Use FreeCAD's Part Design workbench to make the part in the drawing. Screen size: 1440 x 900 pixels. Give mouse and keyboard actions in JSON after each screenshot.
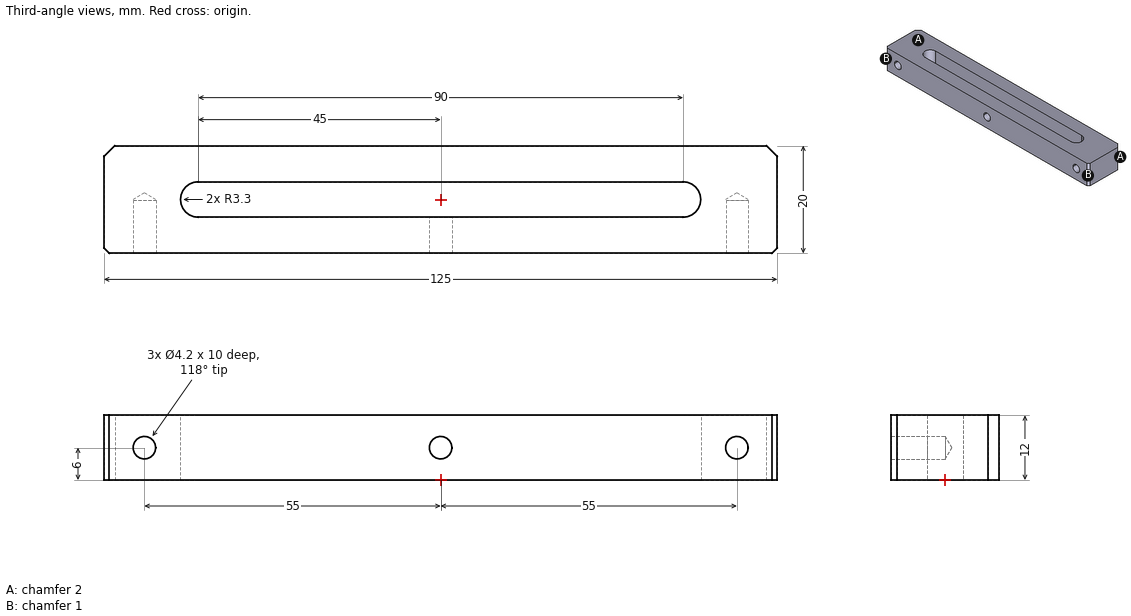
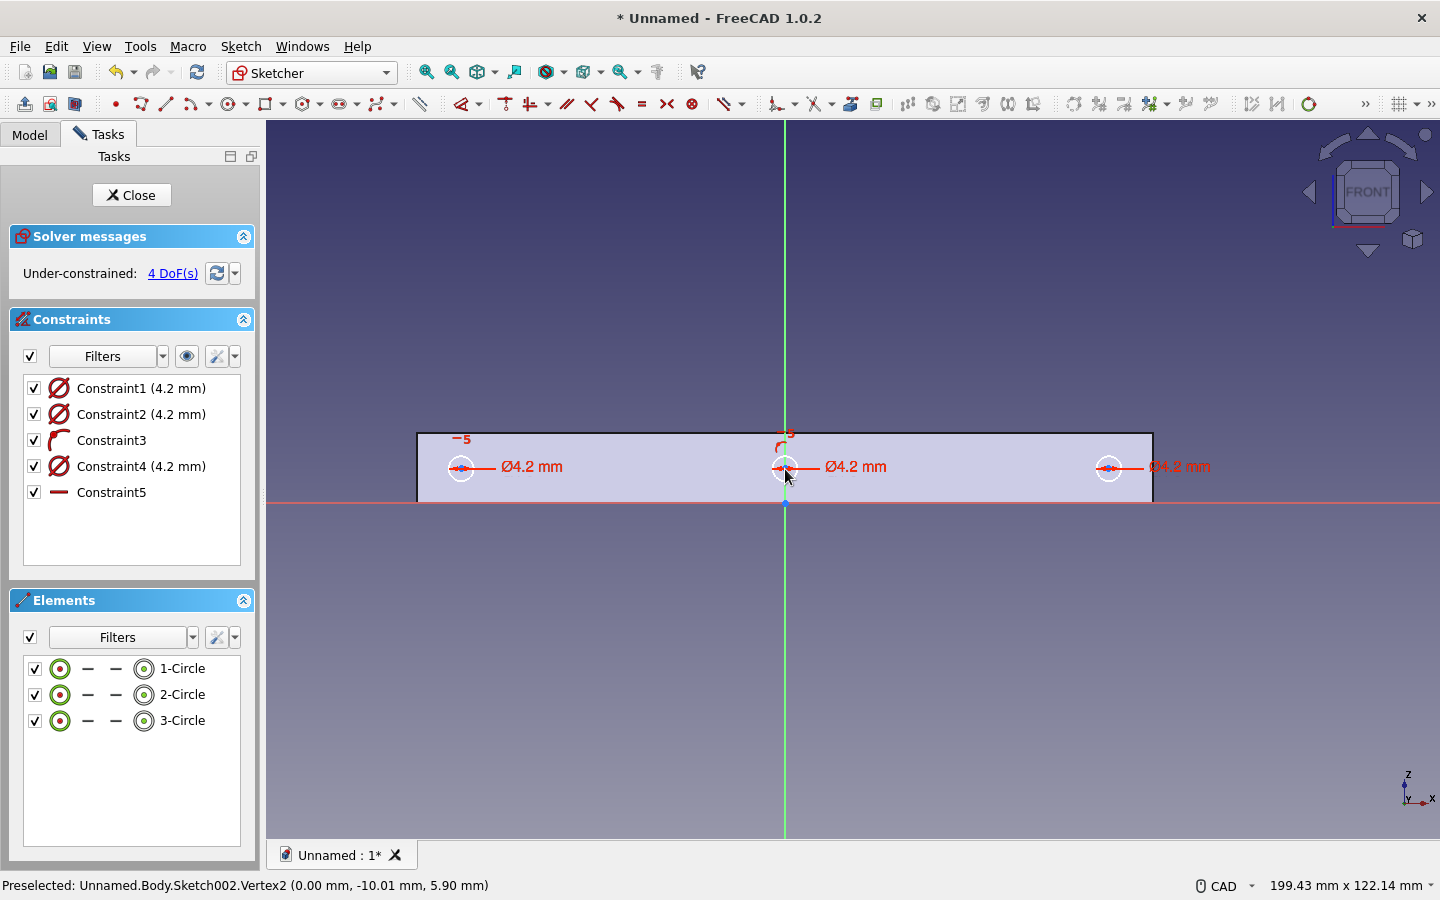
{"action": "left_click", "coordinate": [785, 469]}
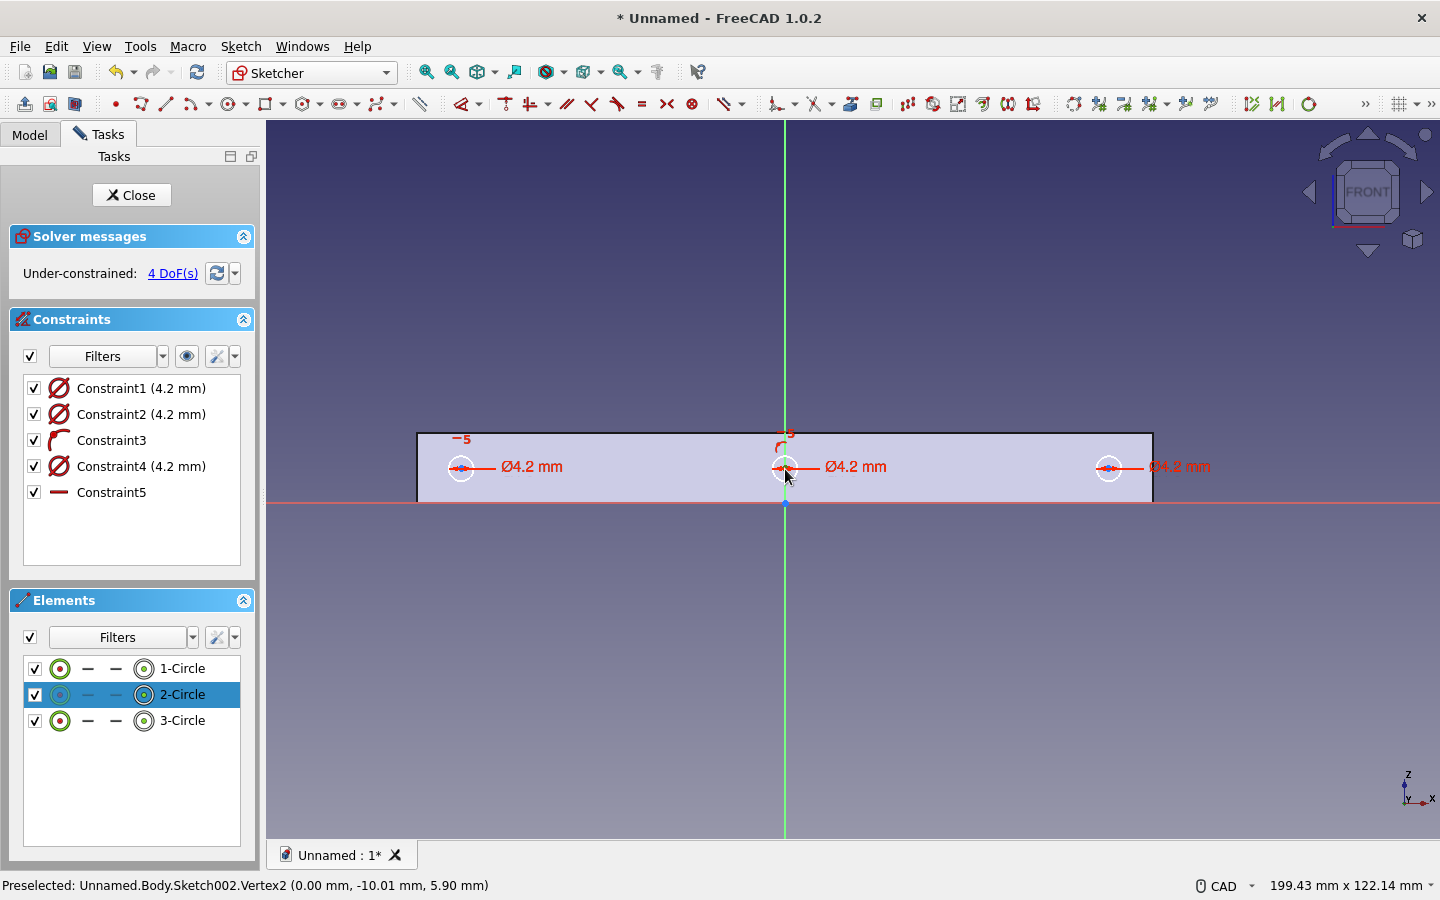
{"action": "left_click", "coordinate": [1109, 469]}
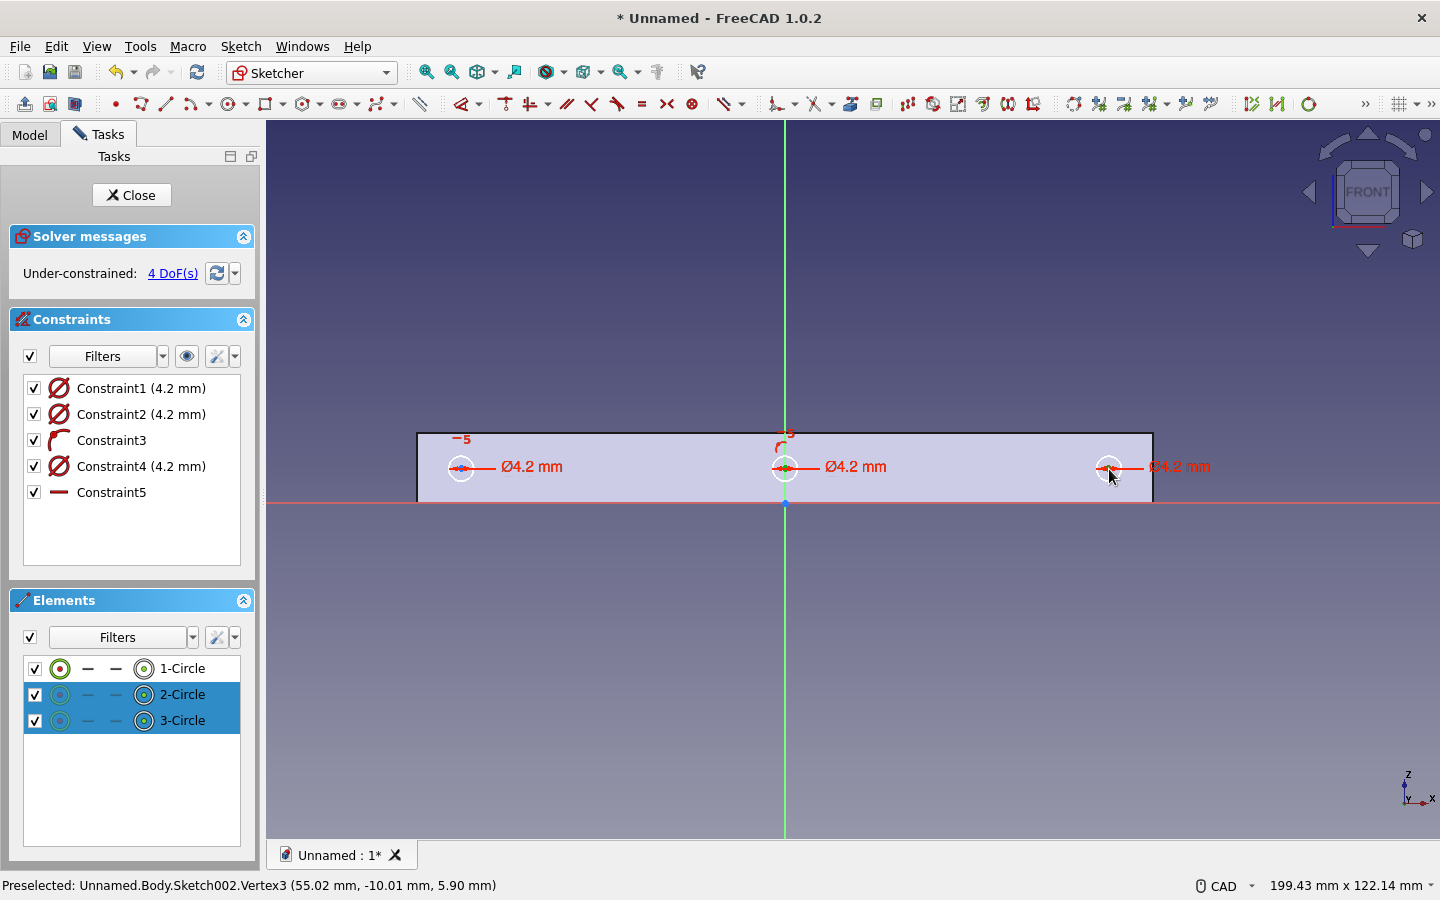
{"action": "key", "text": "h"}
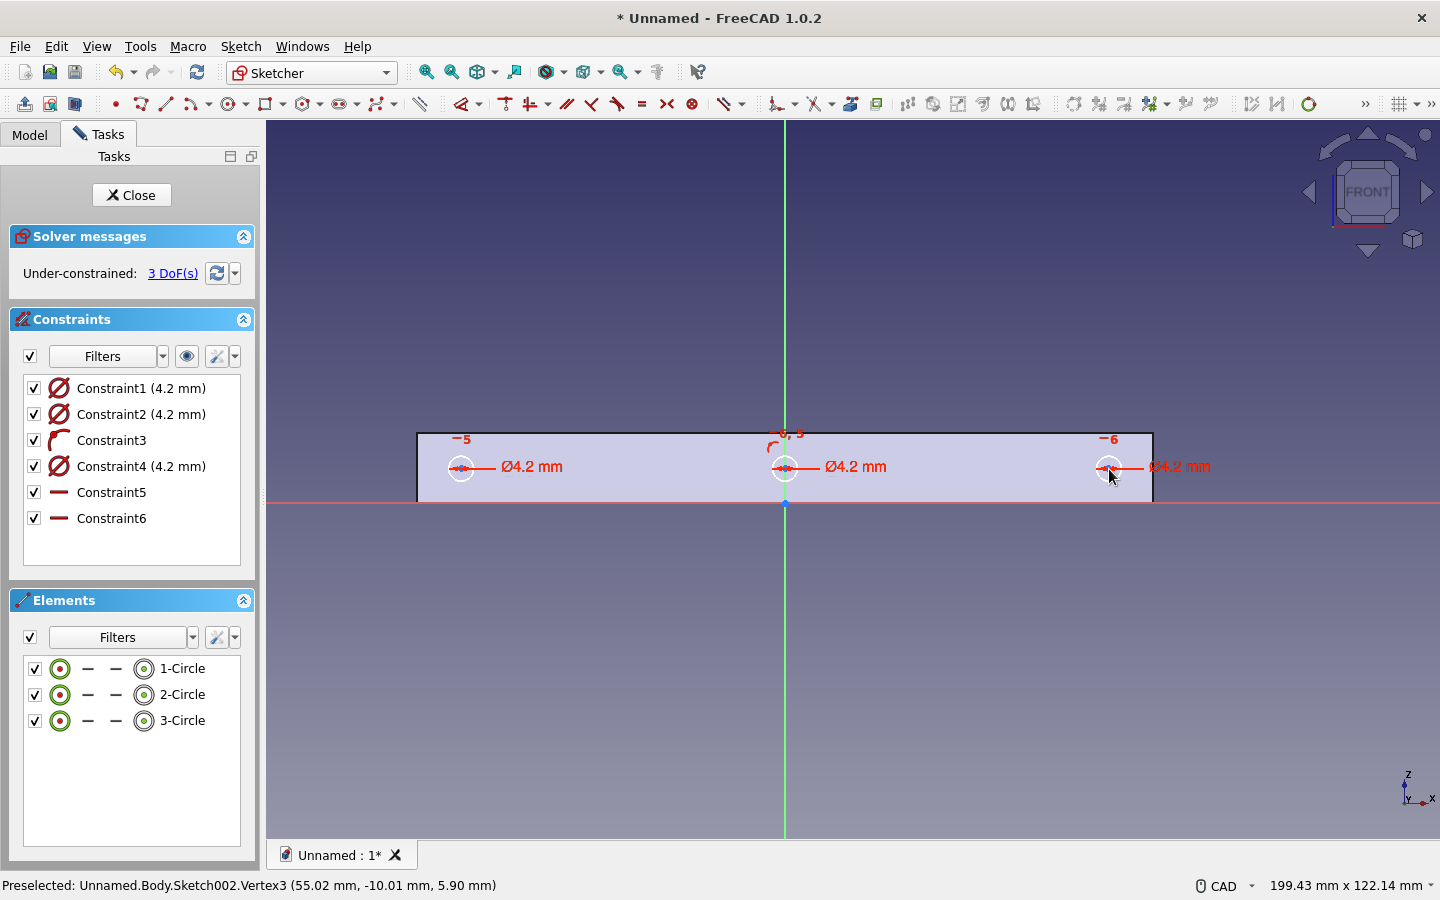
{"action": "key", "text": "d"}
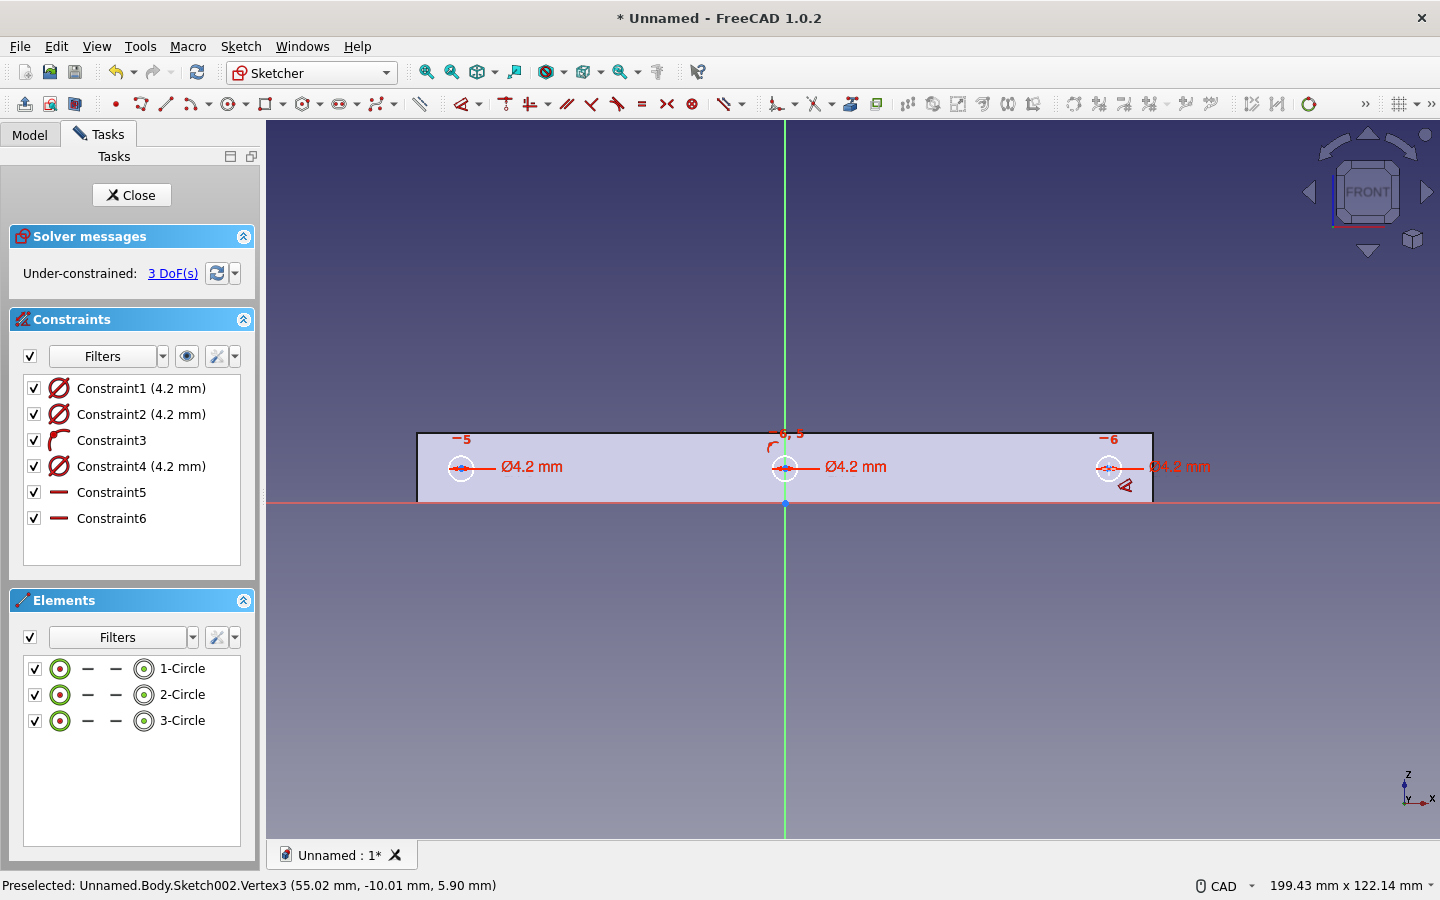
{"action": "left_click", "coordinate": [461, 469]}
{"action": "left_click", "coordinate": [427, 486]}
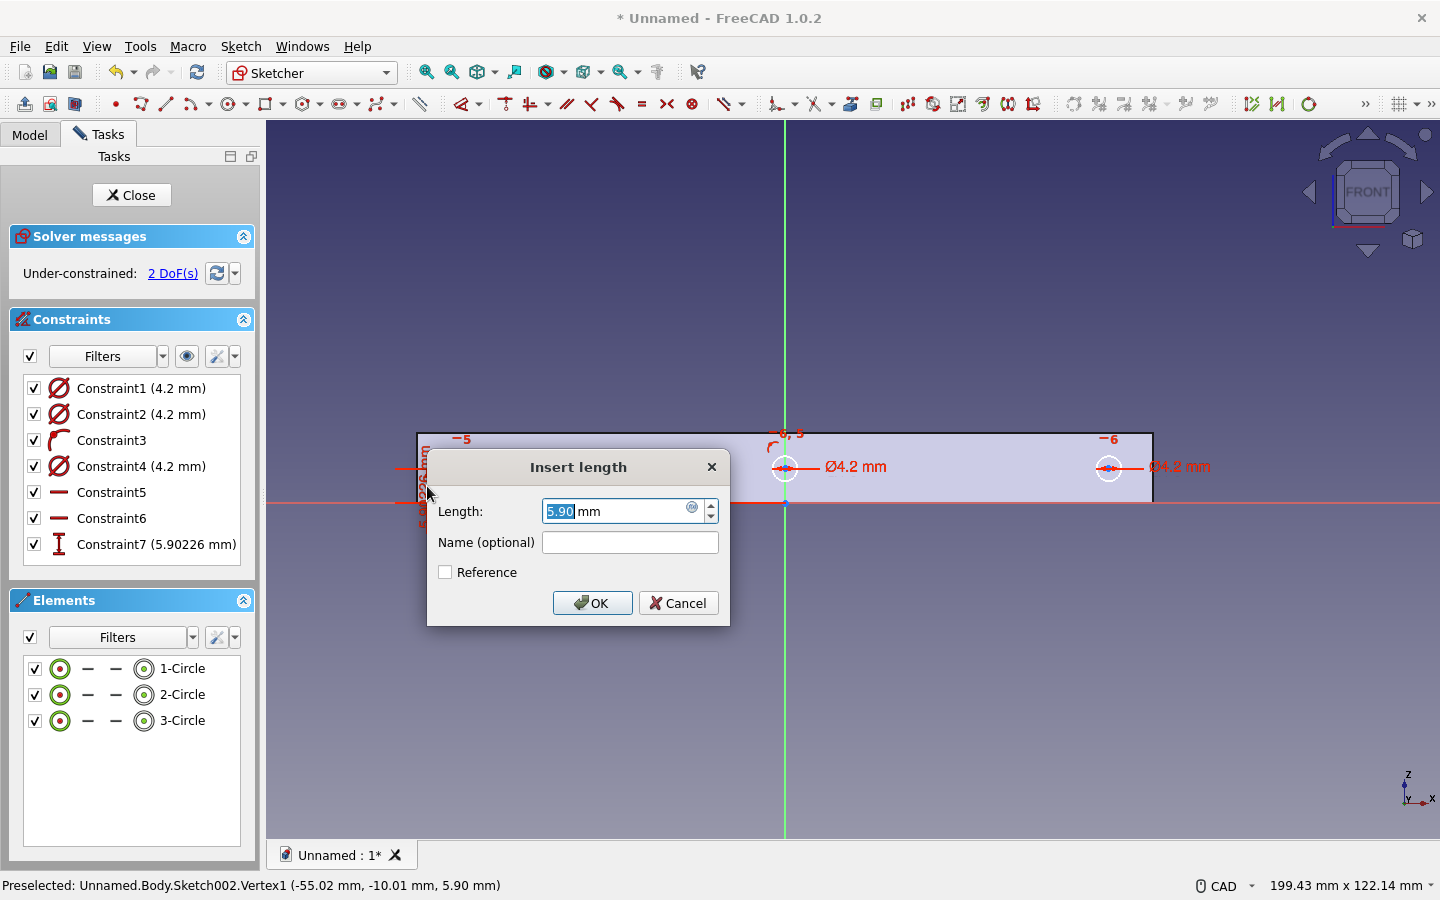
{"action": "type", "text": "6"}
{"action": "key", "text": "Return"}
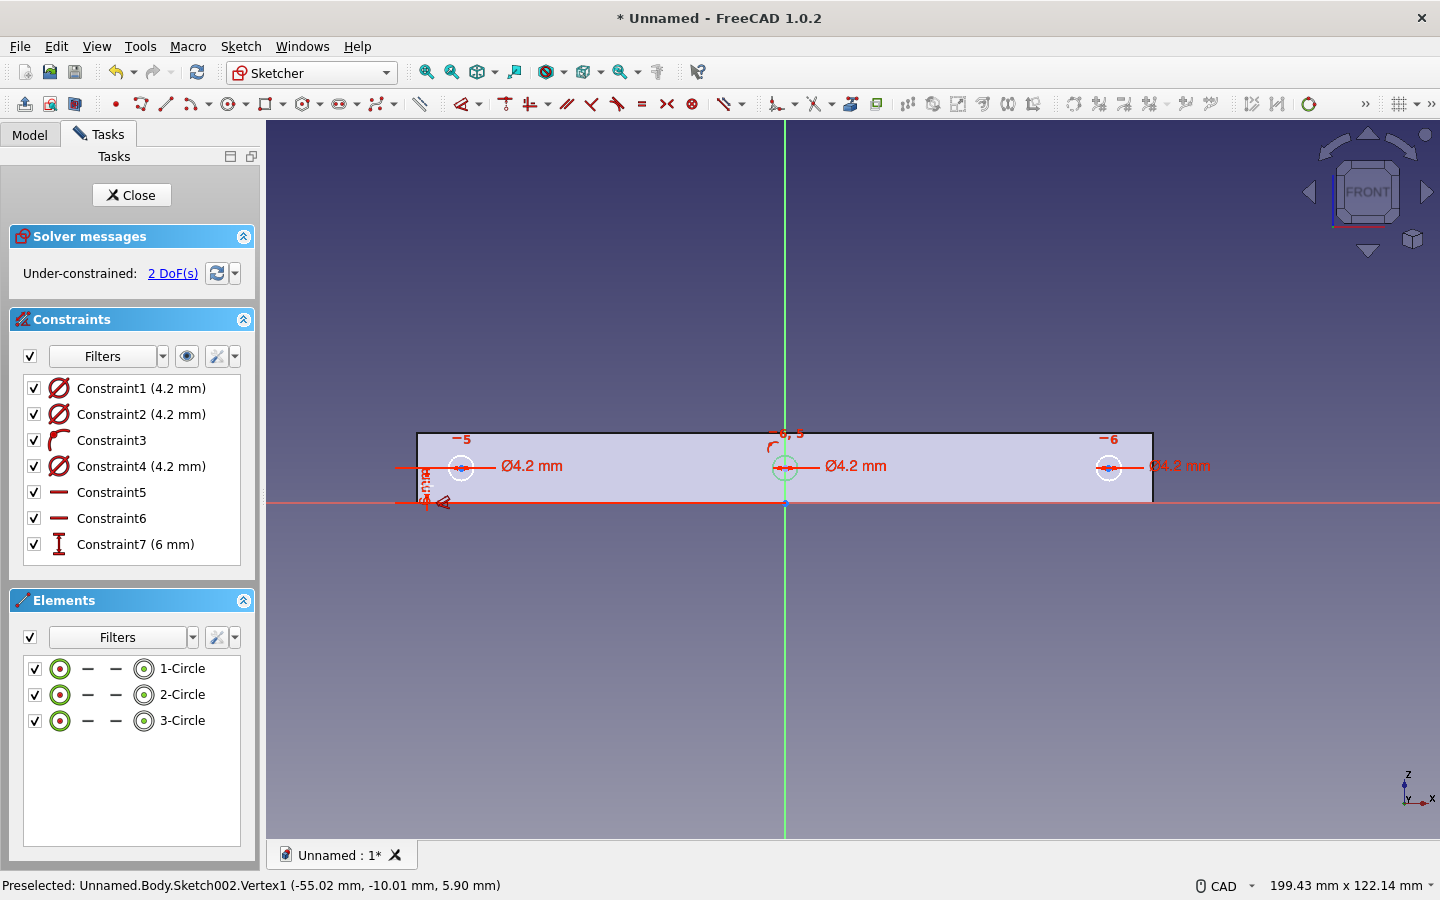
{"action": "left_click", "coordinate": [461, 468]}
{"action": "left_click", "coordinate": [623, 537]}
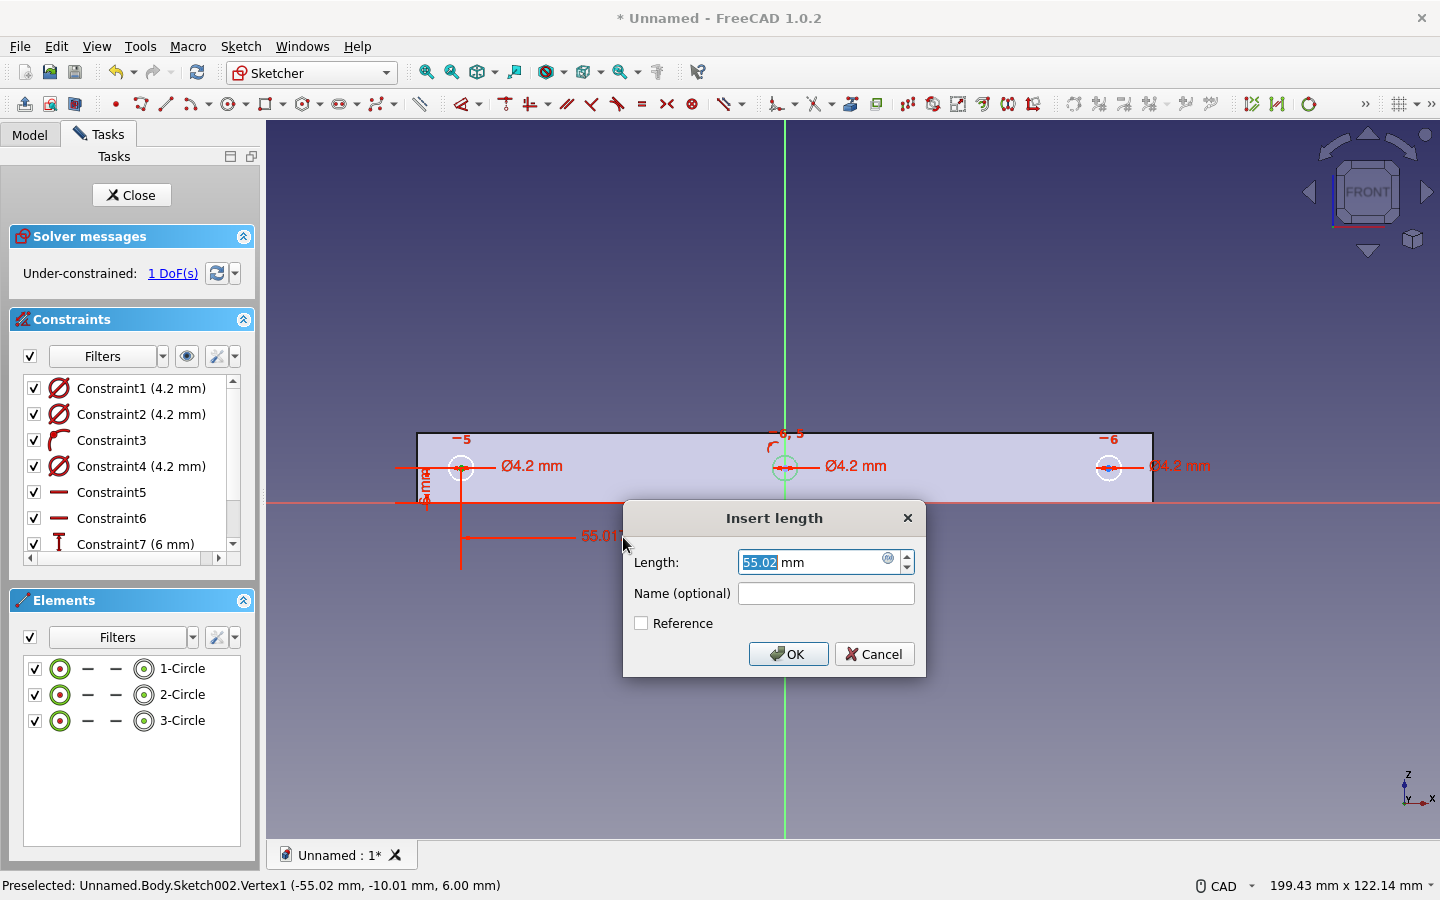
{"action": "type", "text": "55"}
{"action": "key", "text": "Return"}